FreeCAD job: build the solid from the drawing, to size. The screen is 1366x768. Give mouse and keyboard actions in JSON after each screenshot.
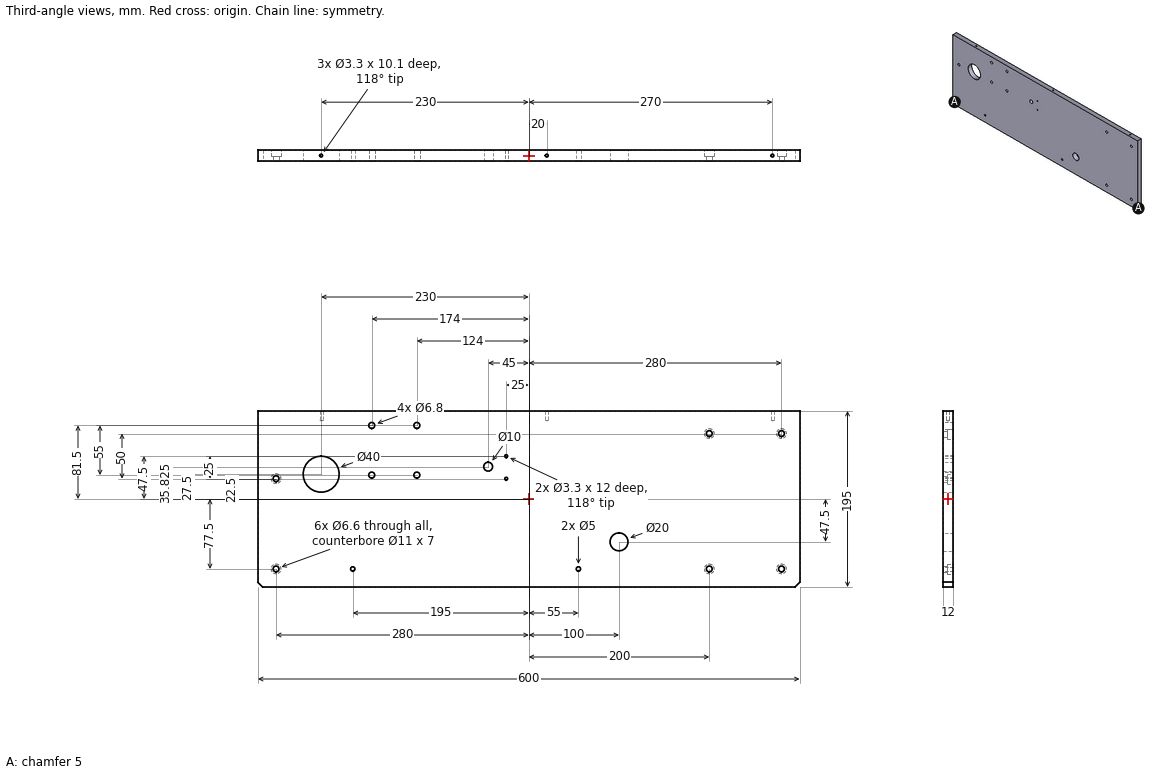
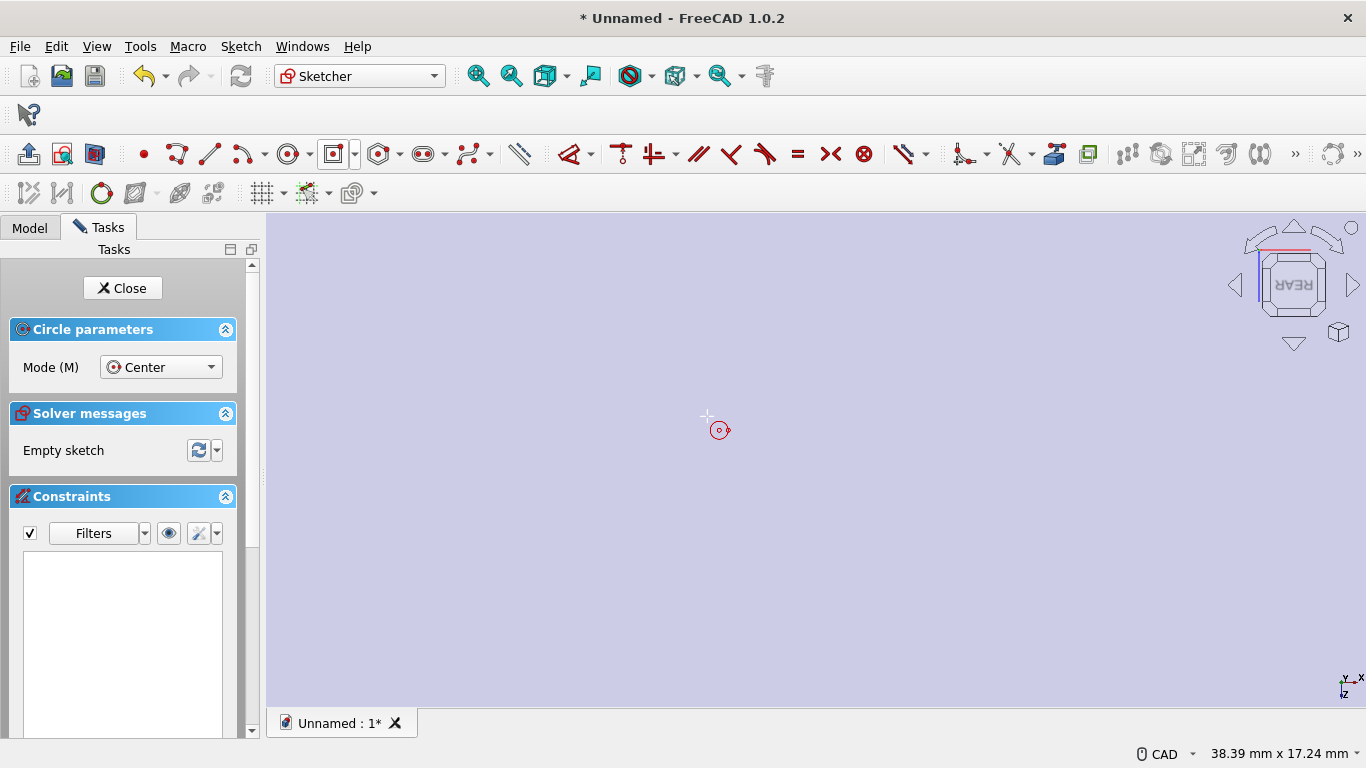
{"action": "left_click", "coordinate": [747, 459]}
{"action": "left_click", "coordinate": [848, 358]}
{"action": "key", "text": "Escape"}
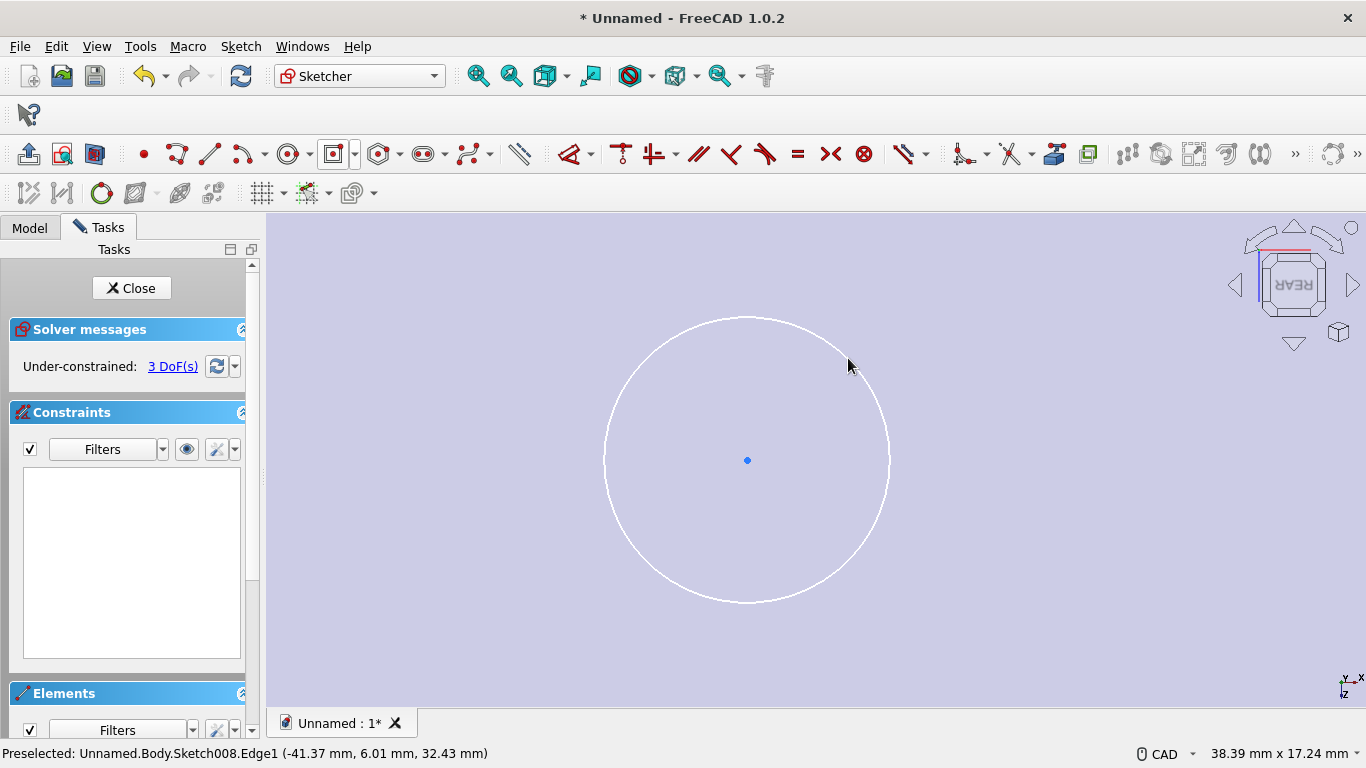
{"action": "key", "text": "d"}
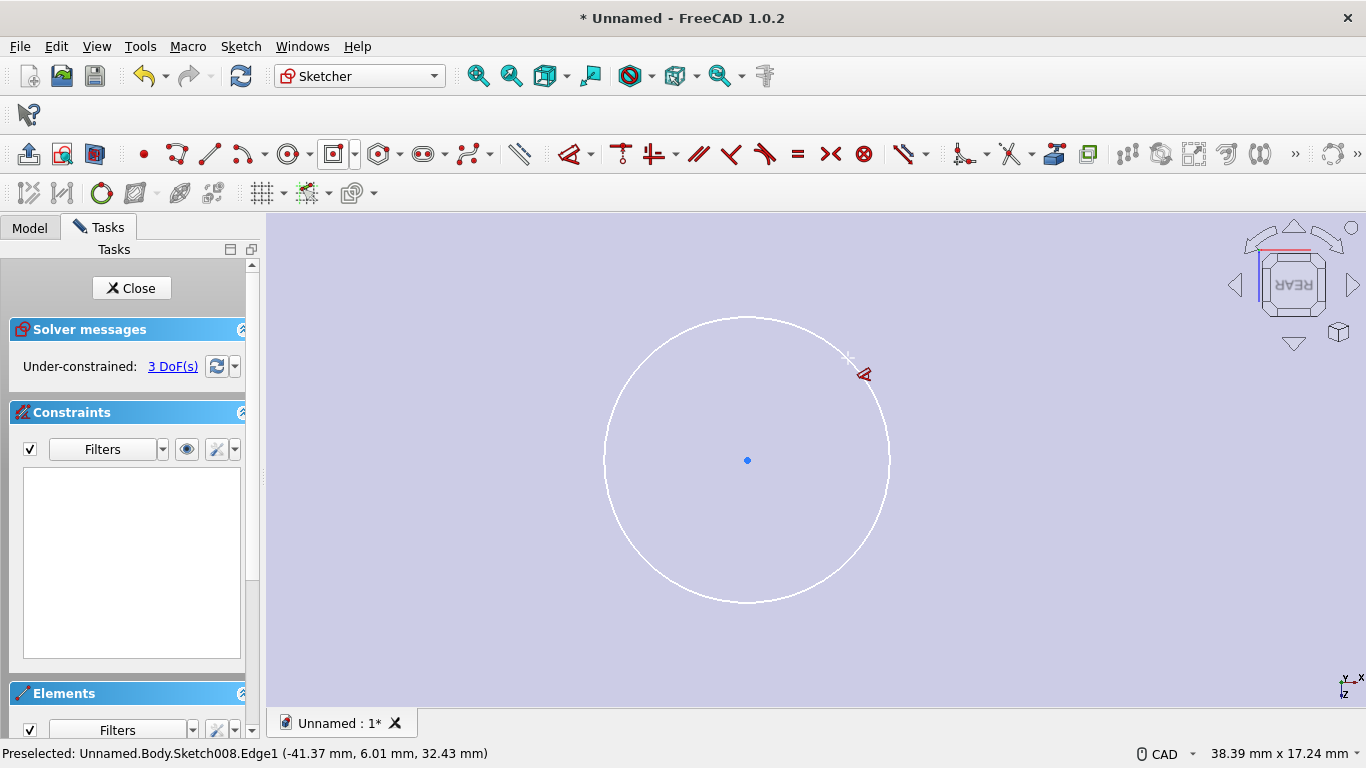
{"action": "left_click", "coordinate": [848, 359]}
{"action": "left_click", "coordinate": [871, 336]}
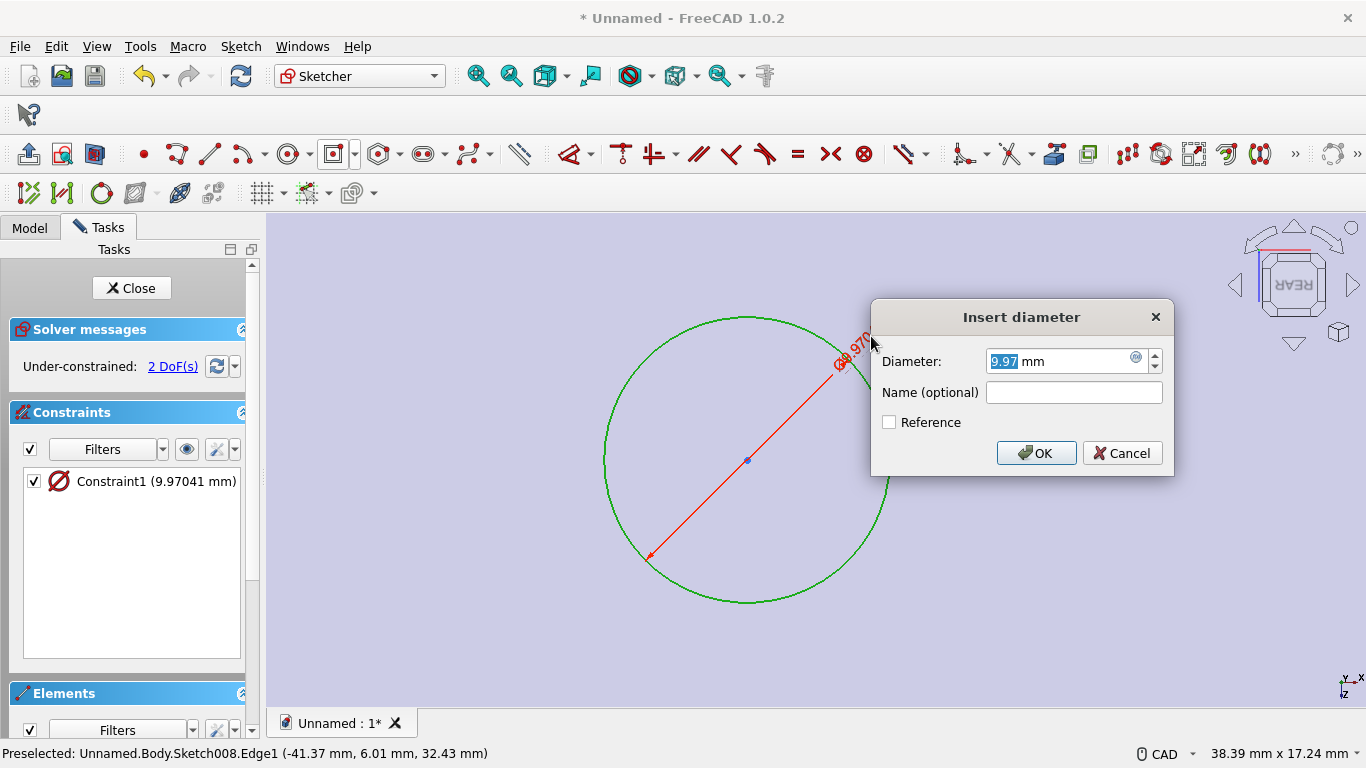
{"action": "type", "text": "10"}
{"action": "key", "text": "Return"}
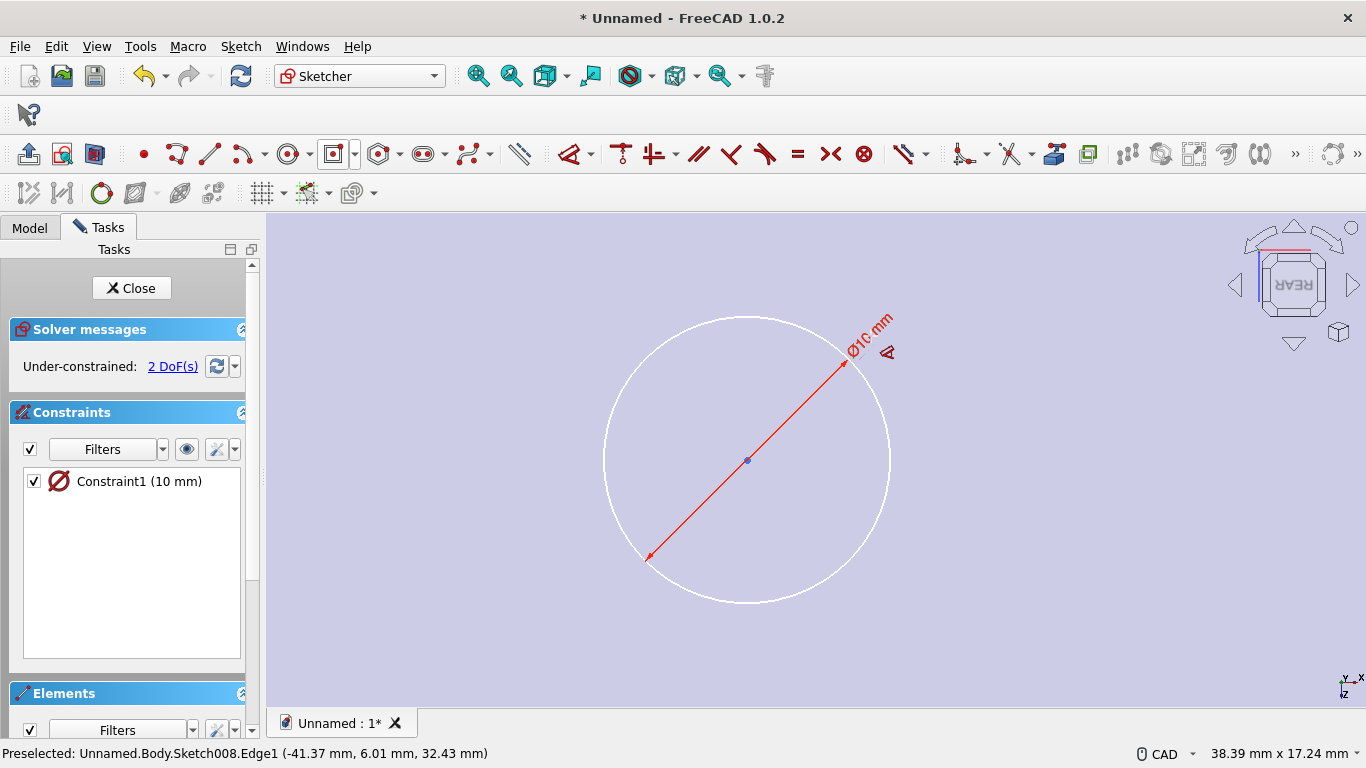
{"action": "left_click", "coordinate": [747, 460]}
{"action": "left_click", "coordinate": [974, 494]}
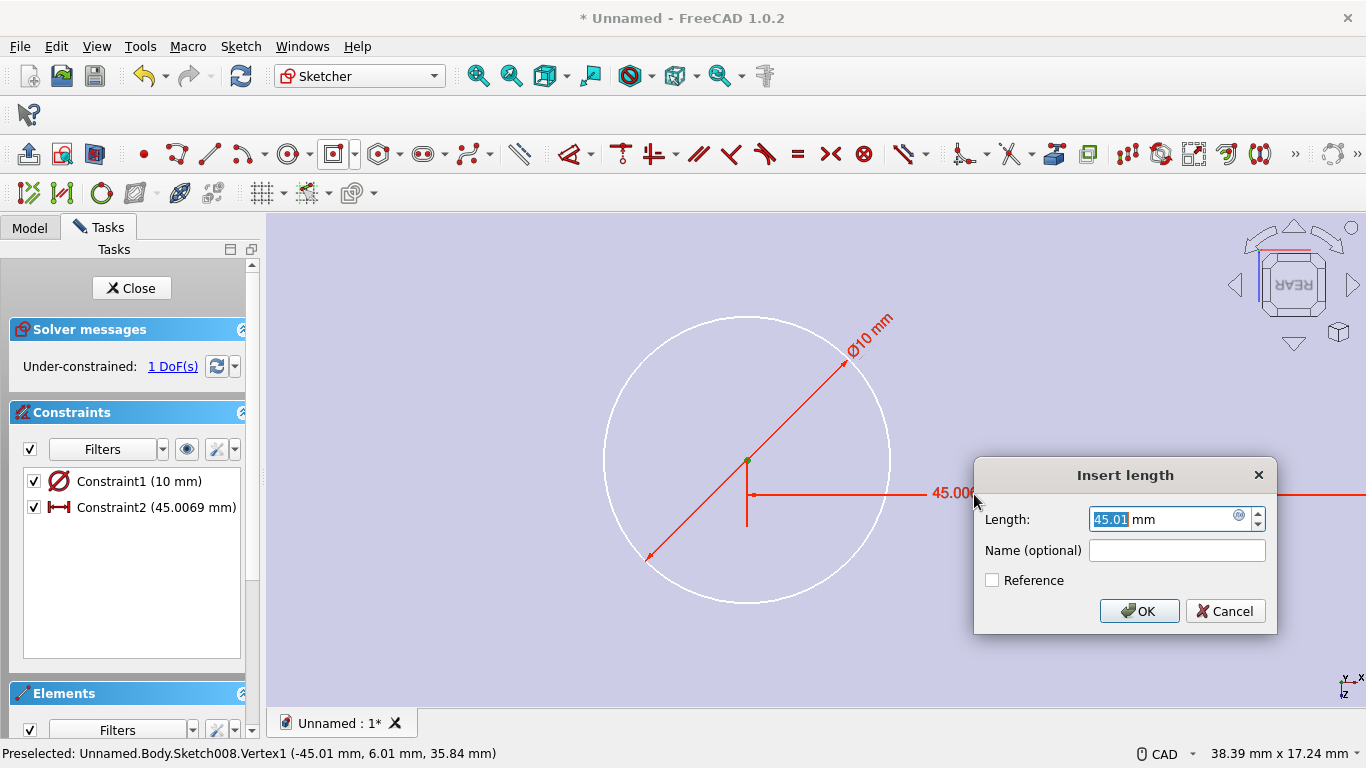
{"action": "type", "text": "45"}
{"action": "key", "text": "Return"}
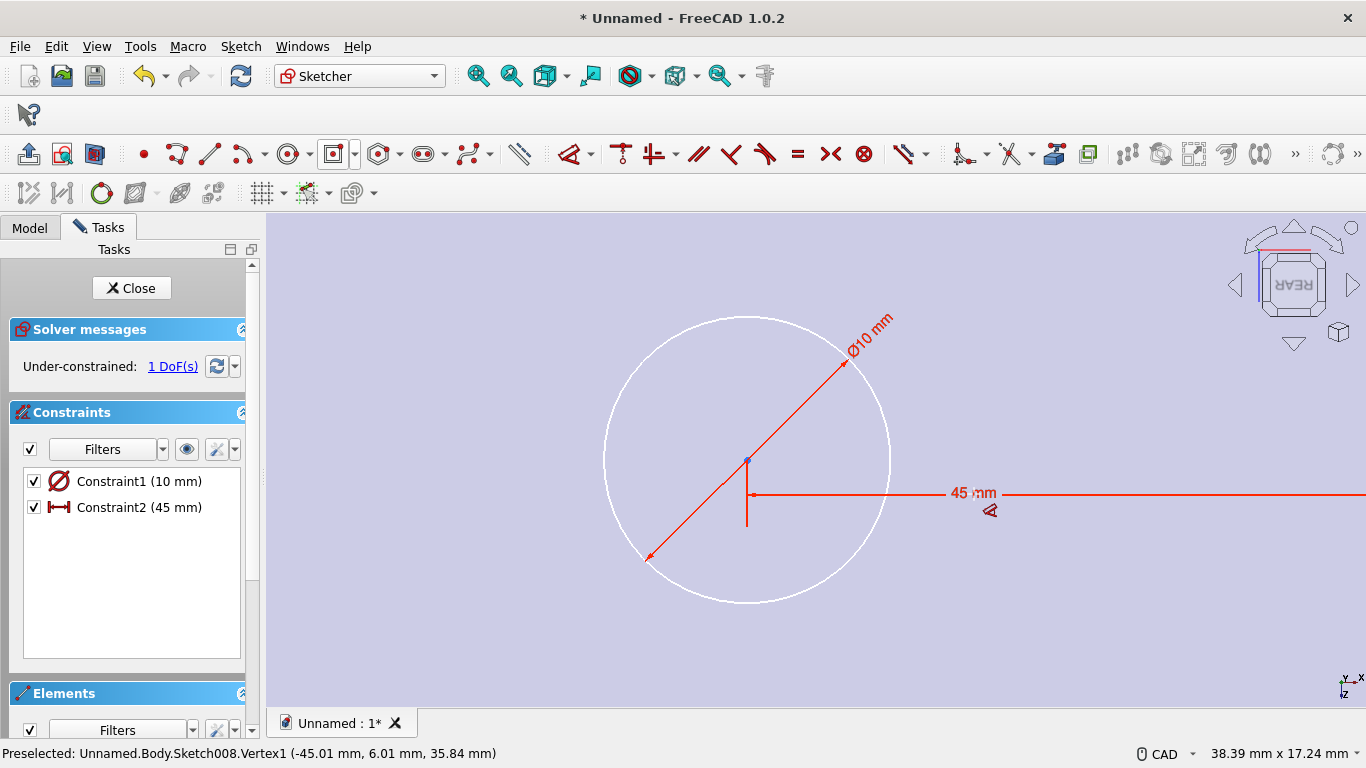
{"action": "left_click", "coordinate": [747, 460]}
{"action": "left_click", "coordinate": [713, 350]}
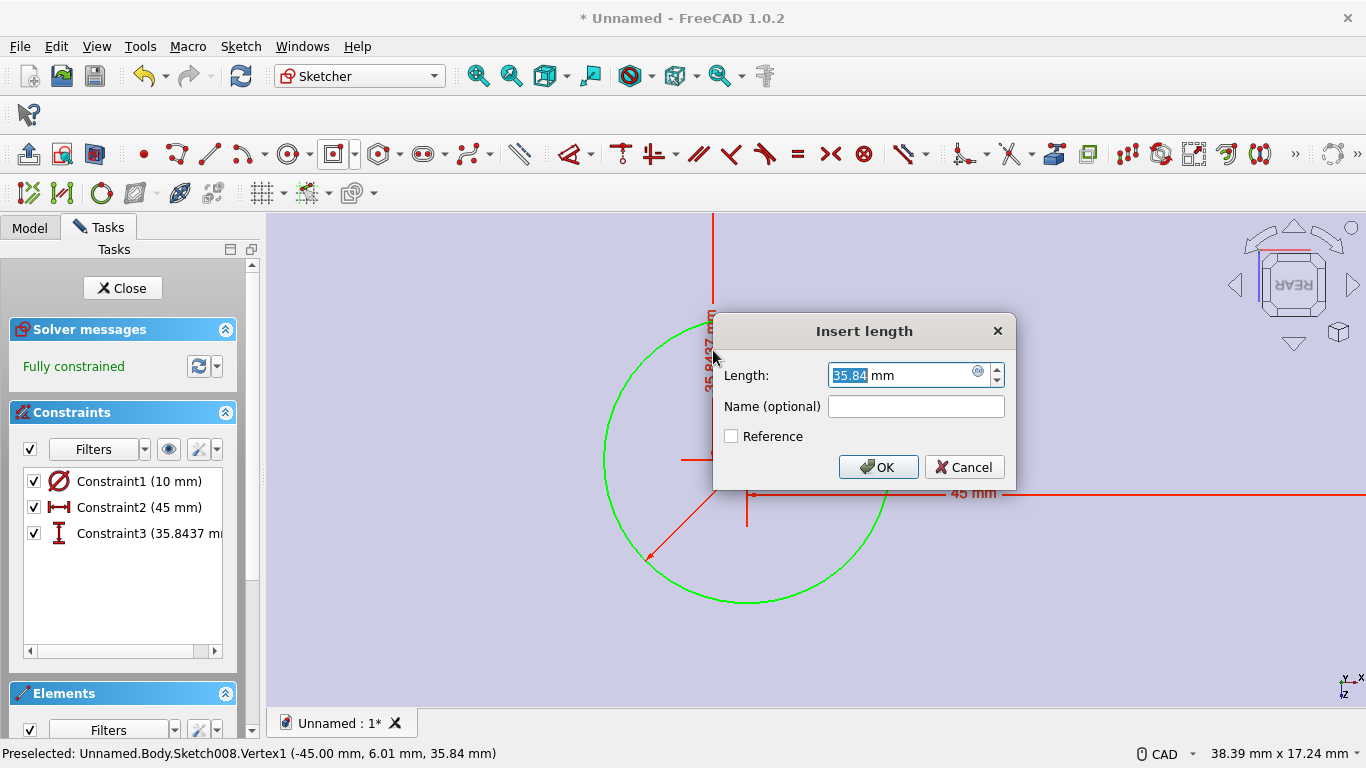
{"action": "type", "text": "35.825"}
{"action": "key", "text": "Return"}
{"action": "key", "text": "Escape"}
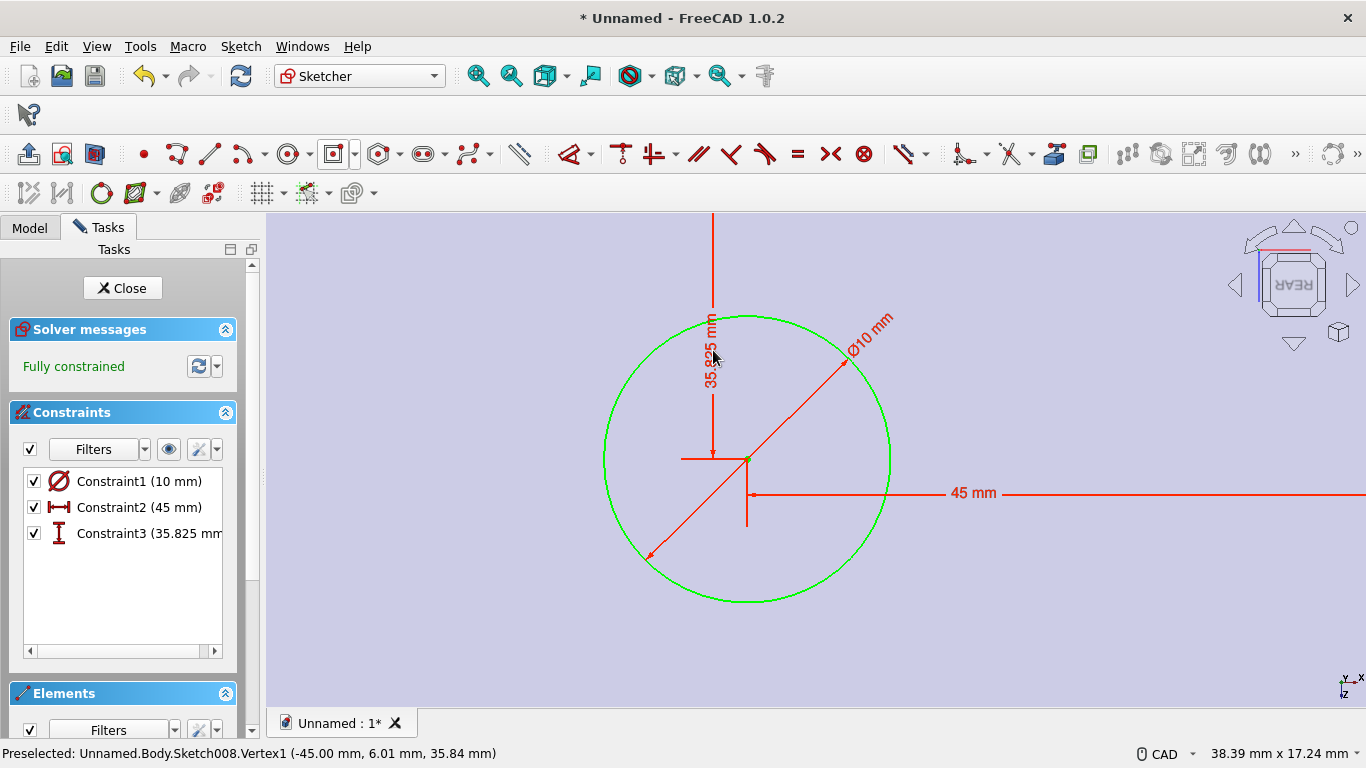
{"action": "left_click", "coordinate": [123, 288]}